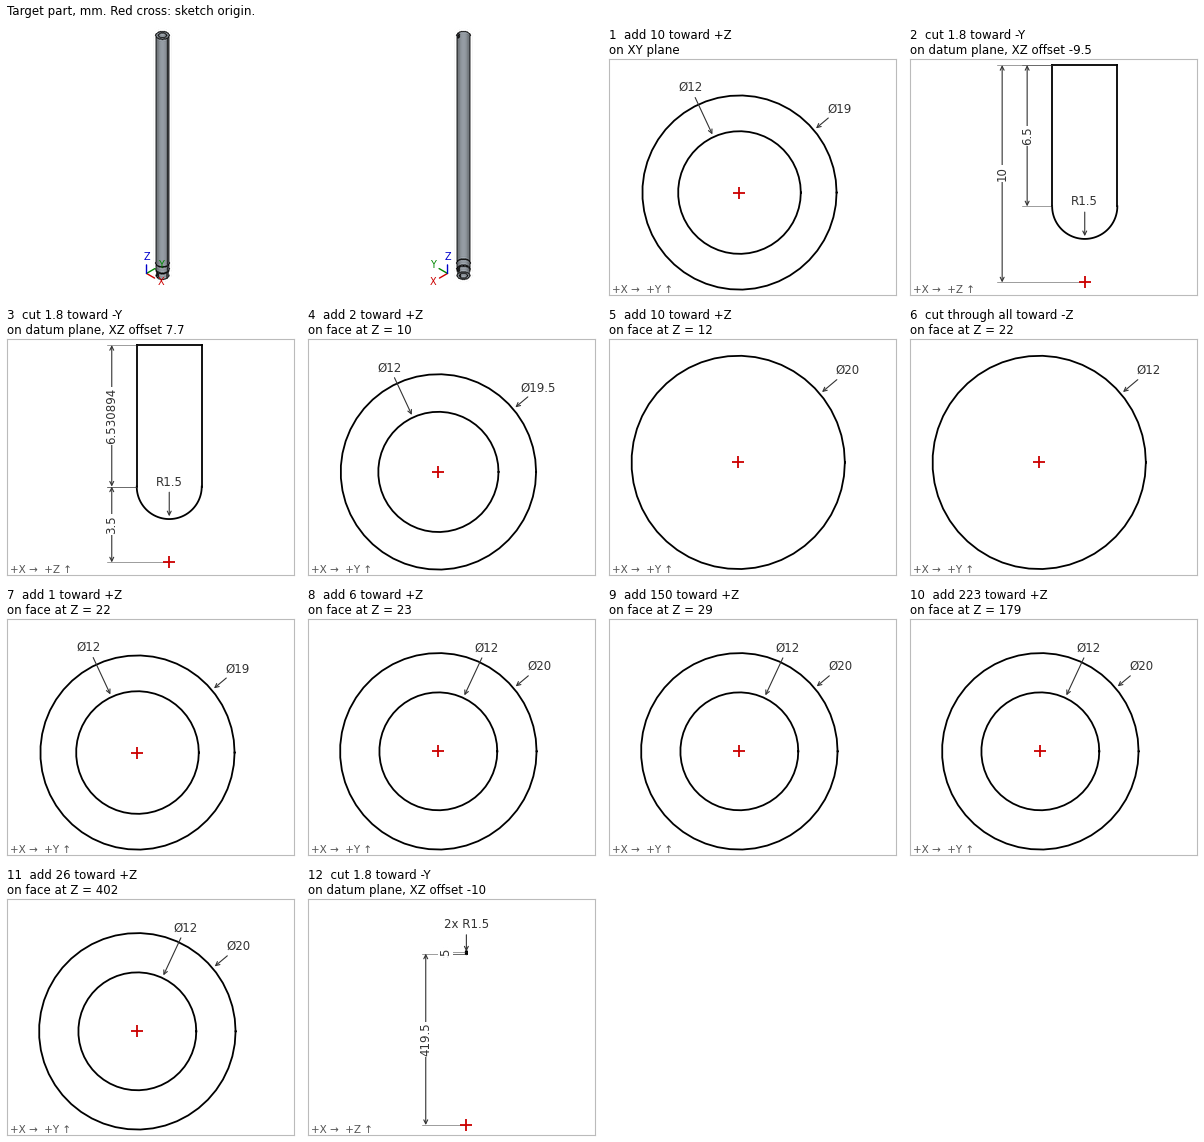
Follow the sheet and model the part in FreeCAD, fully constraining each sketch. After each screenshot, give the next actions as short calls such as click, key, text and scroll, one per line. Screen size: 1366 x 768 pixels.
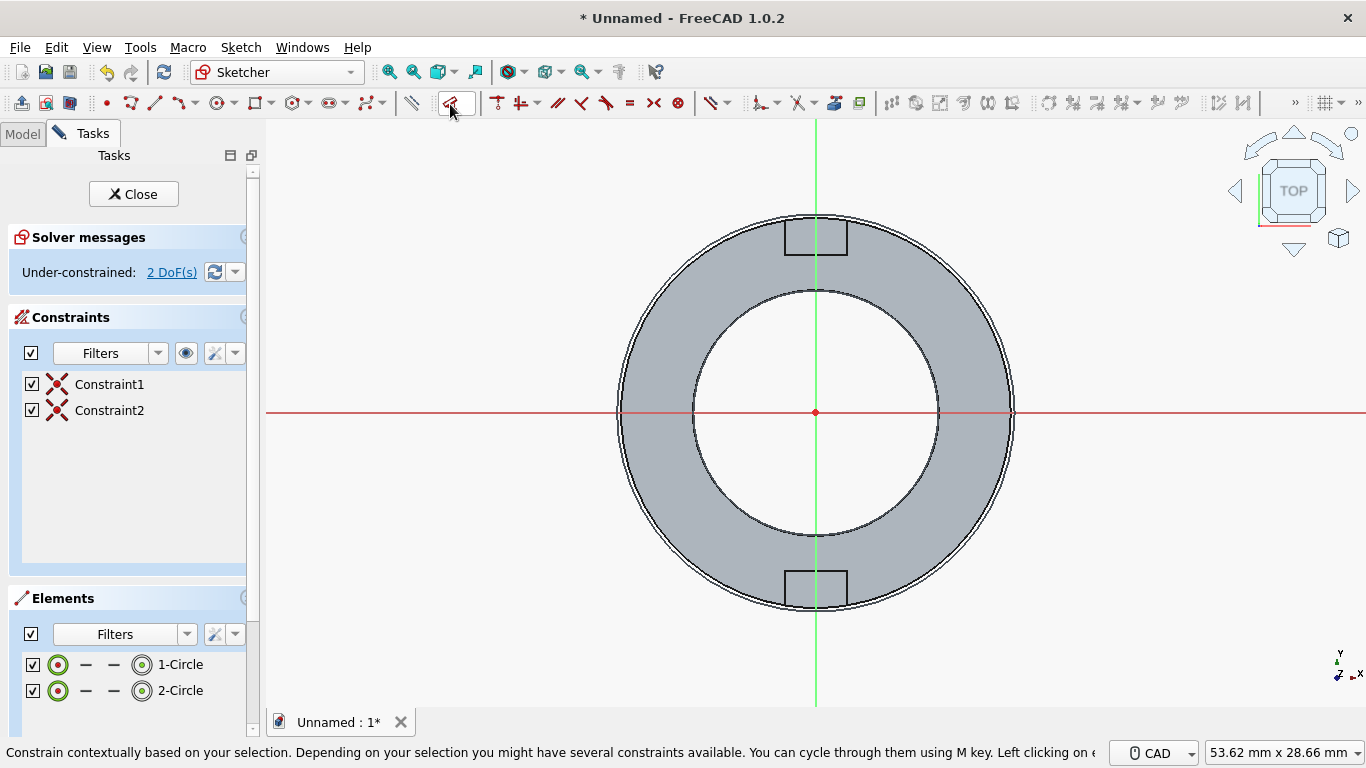
click(956, 272)
click(979, 249)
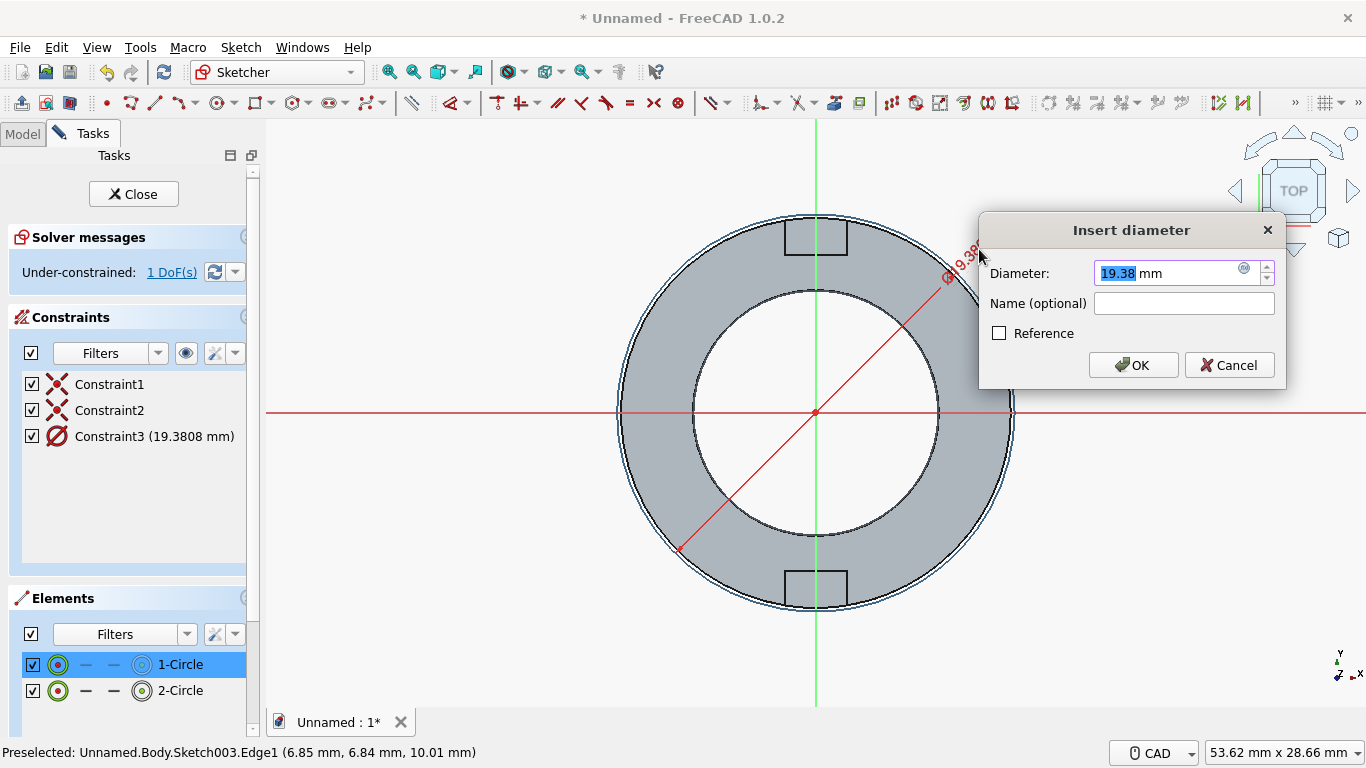
text(19.5)
key(Return)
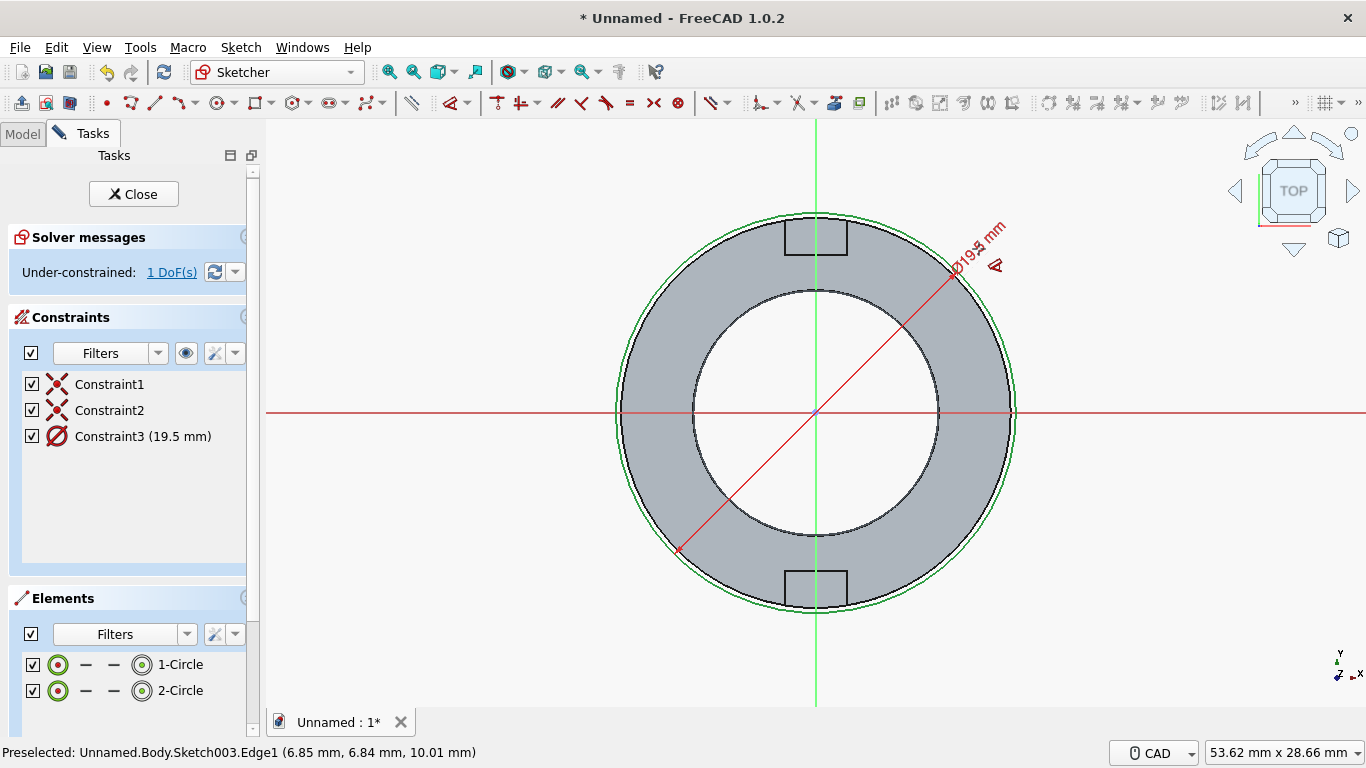
click(902, 326)
click(925, 303)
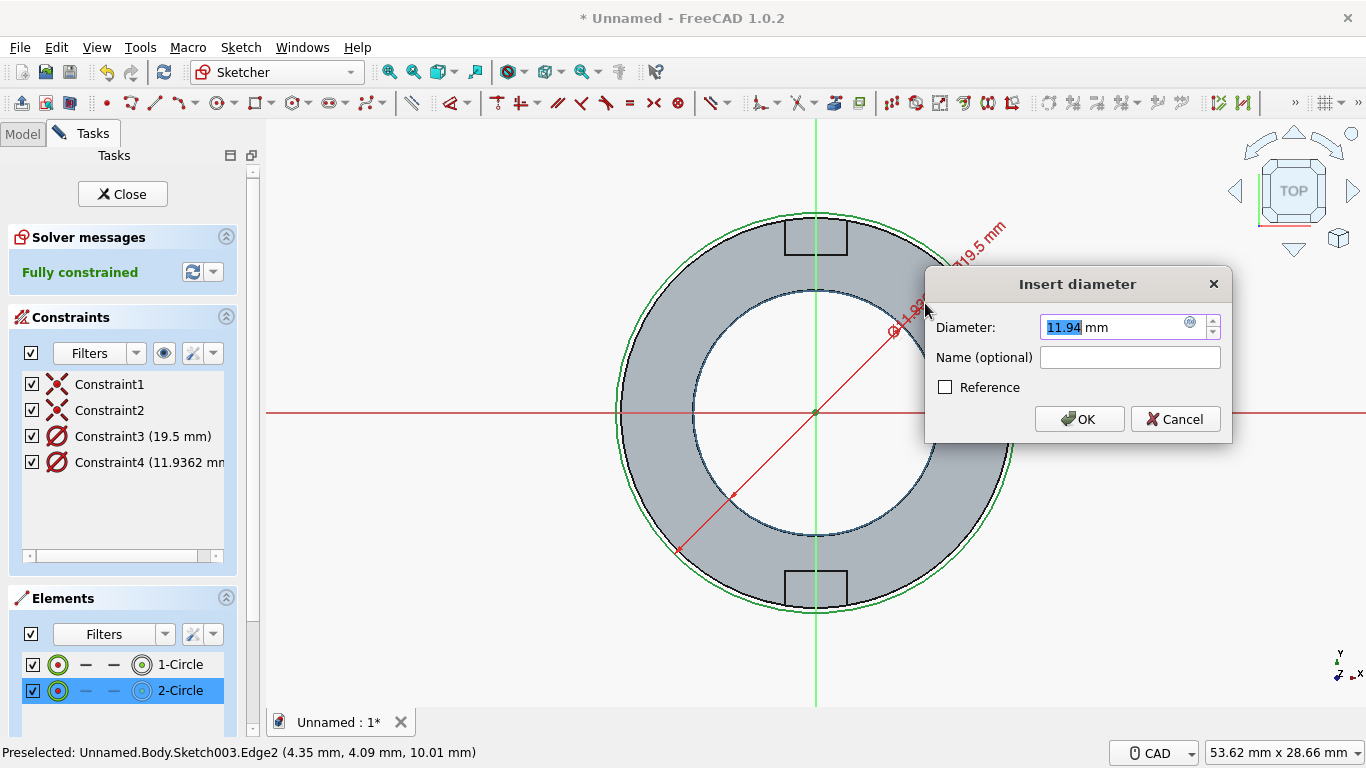
text(12)
key(Return)
key(Escape)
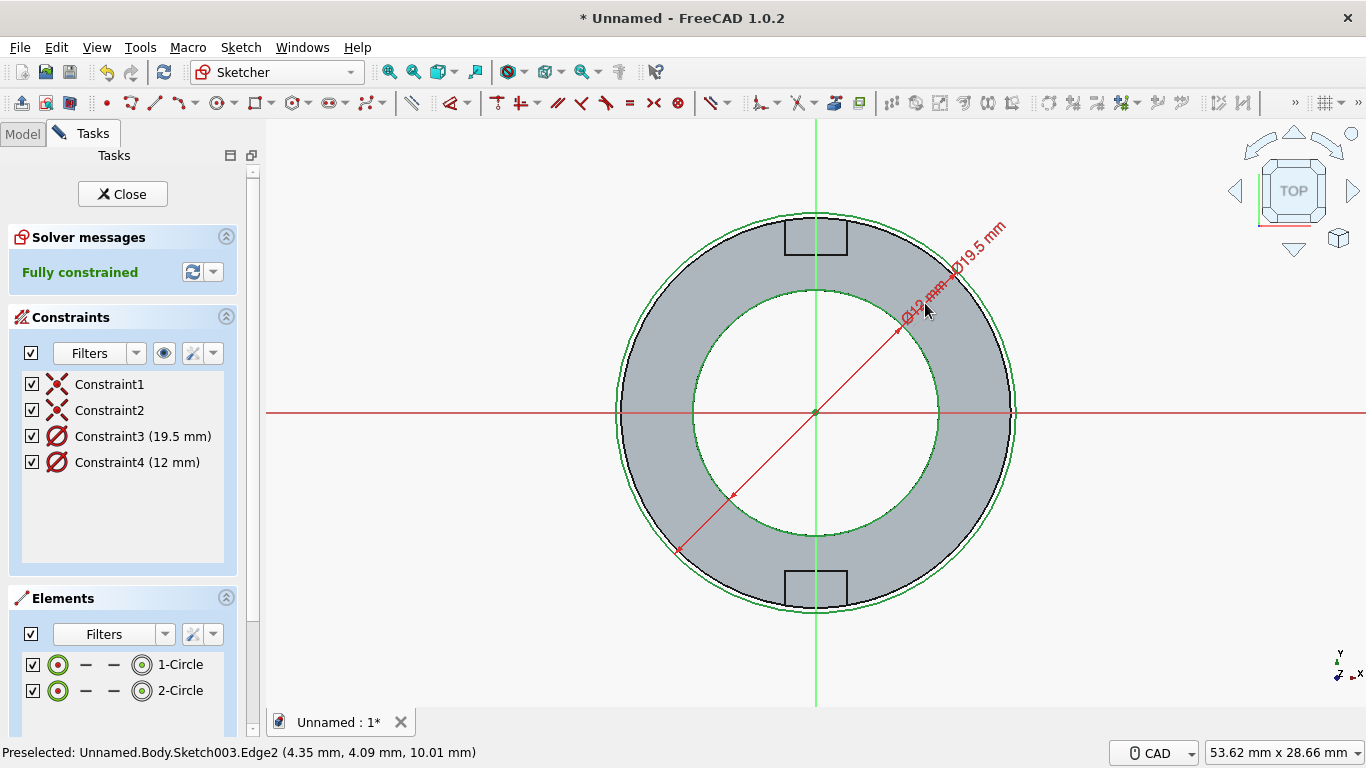
click(123, 194)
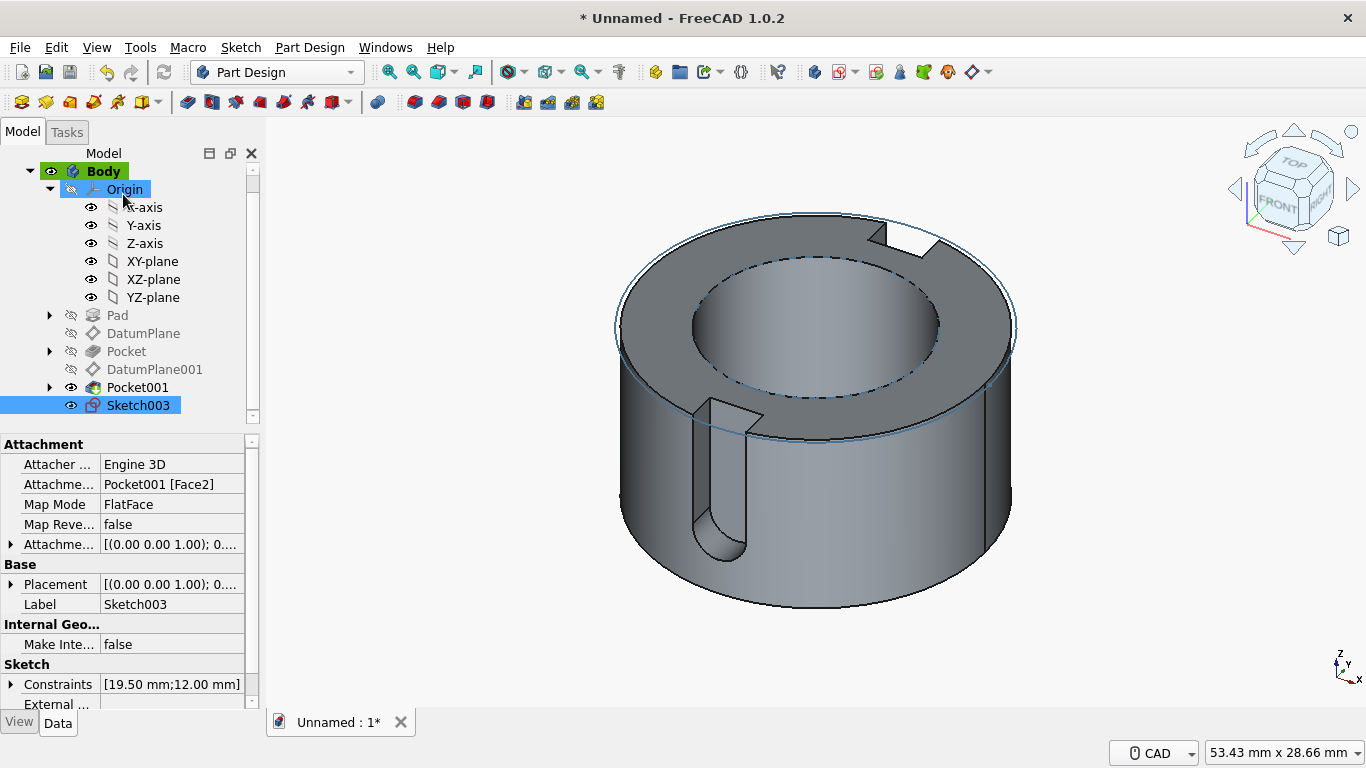
click(22, 102)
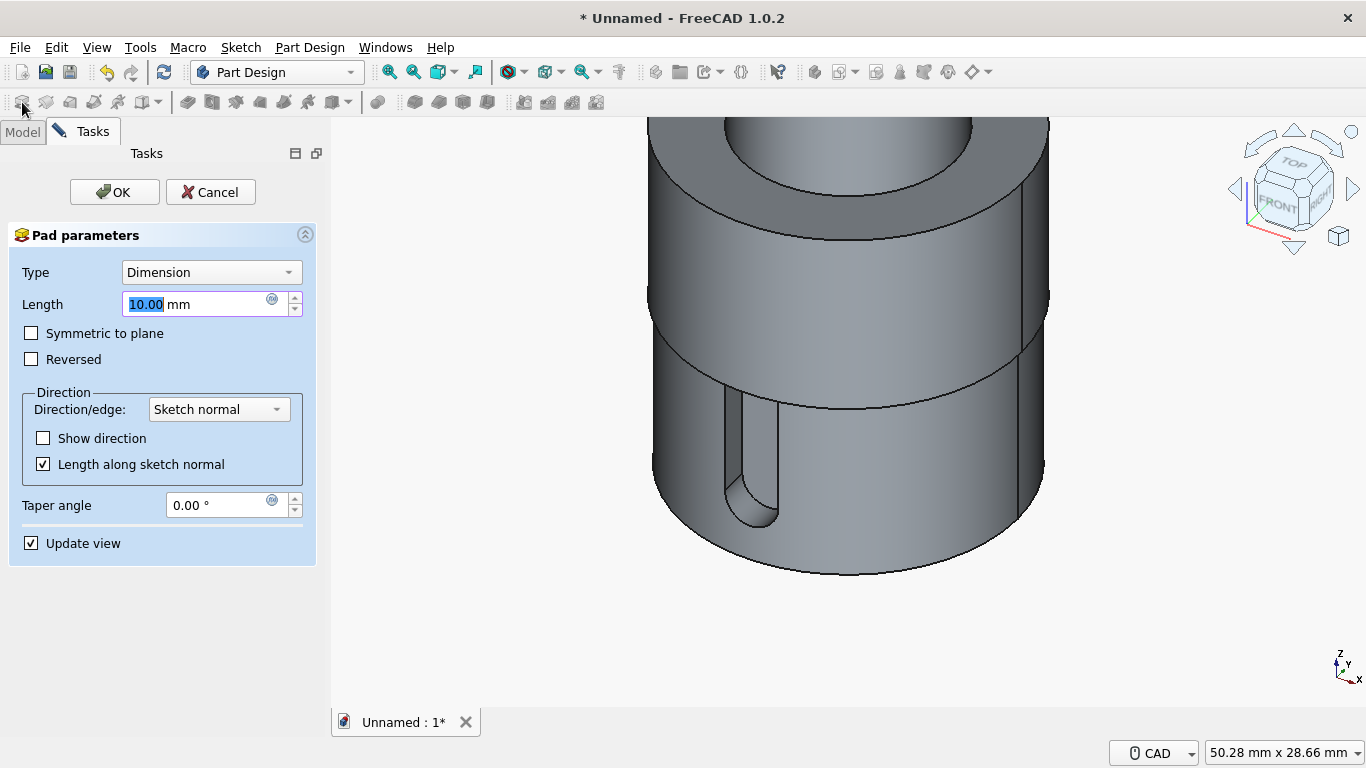
text(2)
key(Tab)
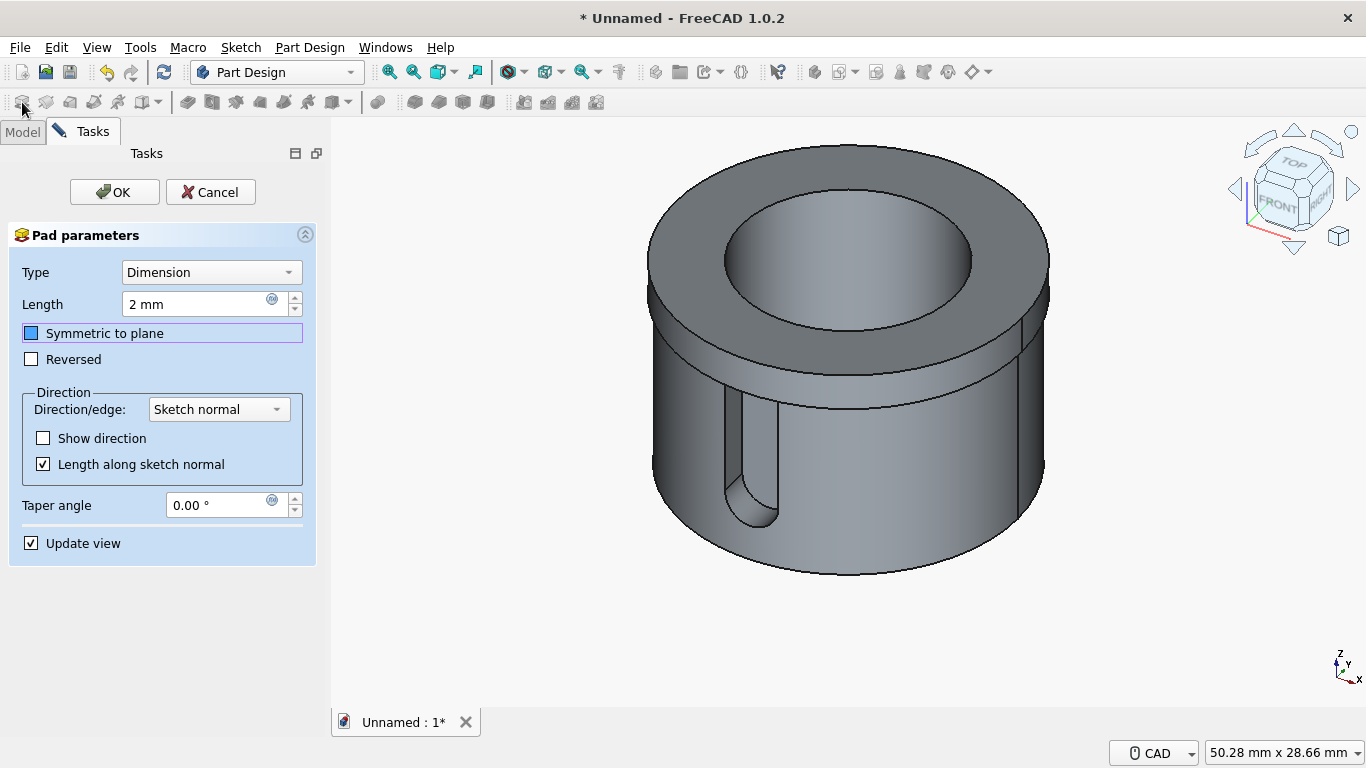
click(115, 192)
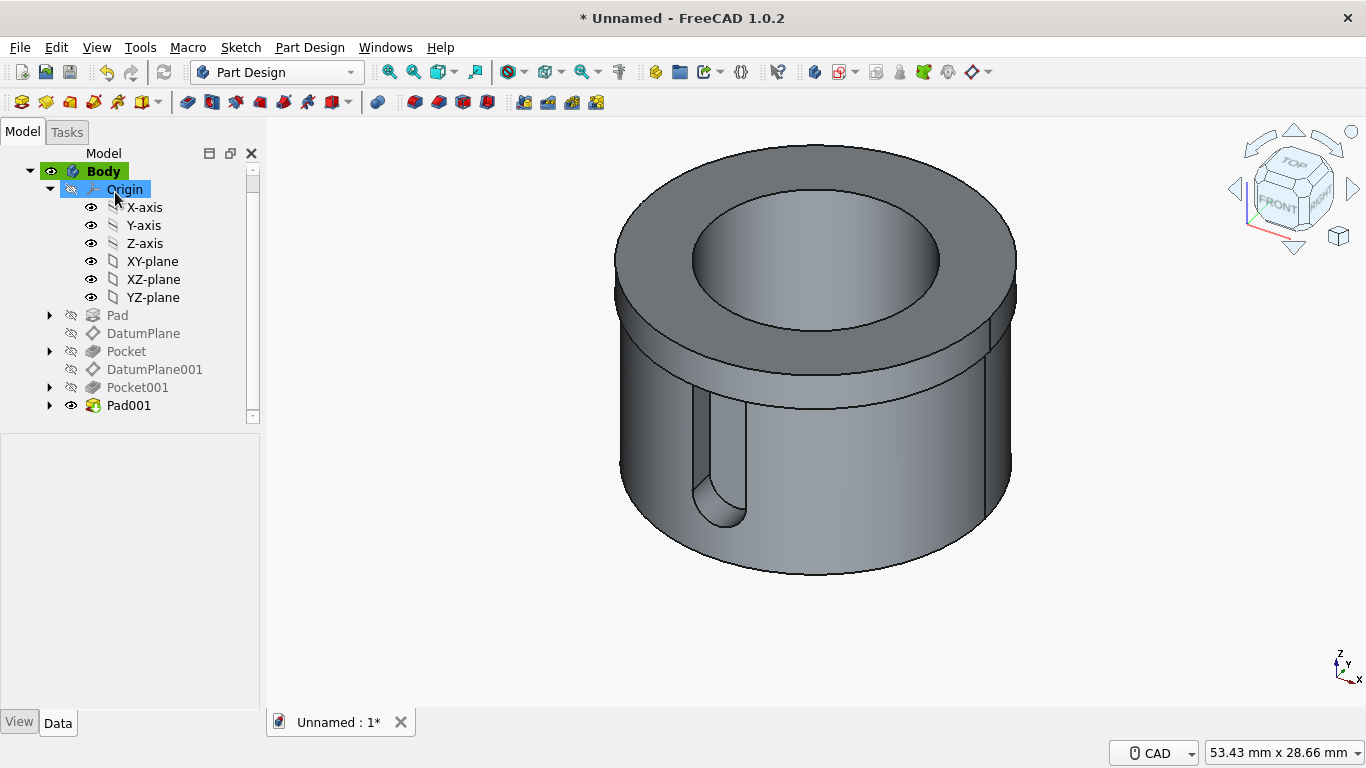
click(390, 72)